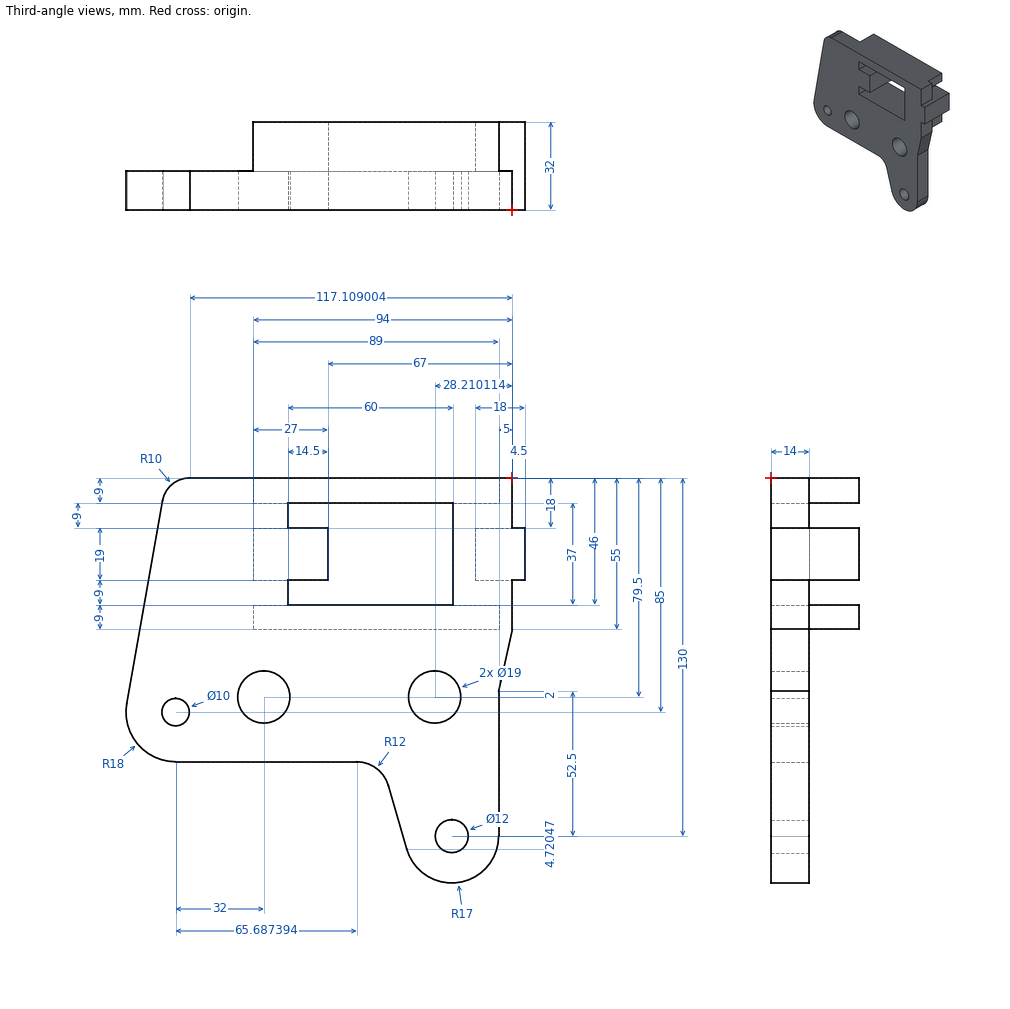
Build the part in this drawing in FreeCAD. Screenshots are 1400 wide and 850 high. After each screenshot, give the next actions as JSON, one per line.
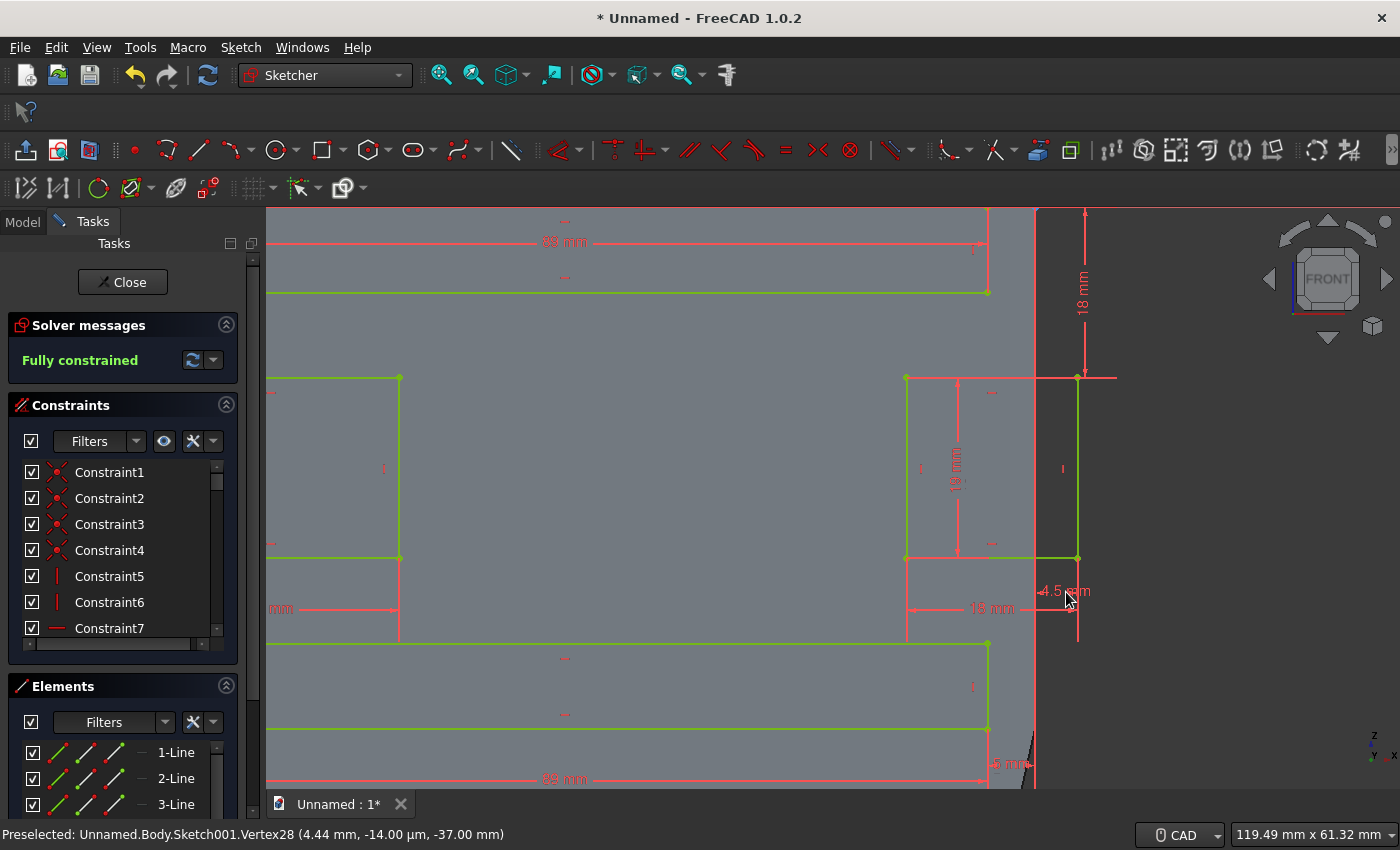
{"action": "left_click", "coordinate": [123, 282]}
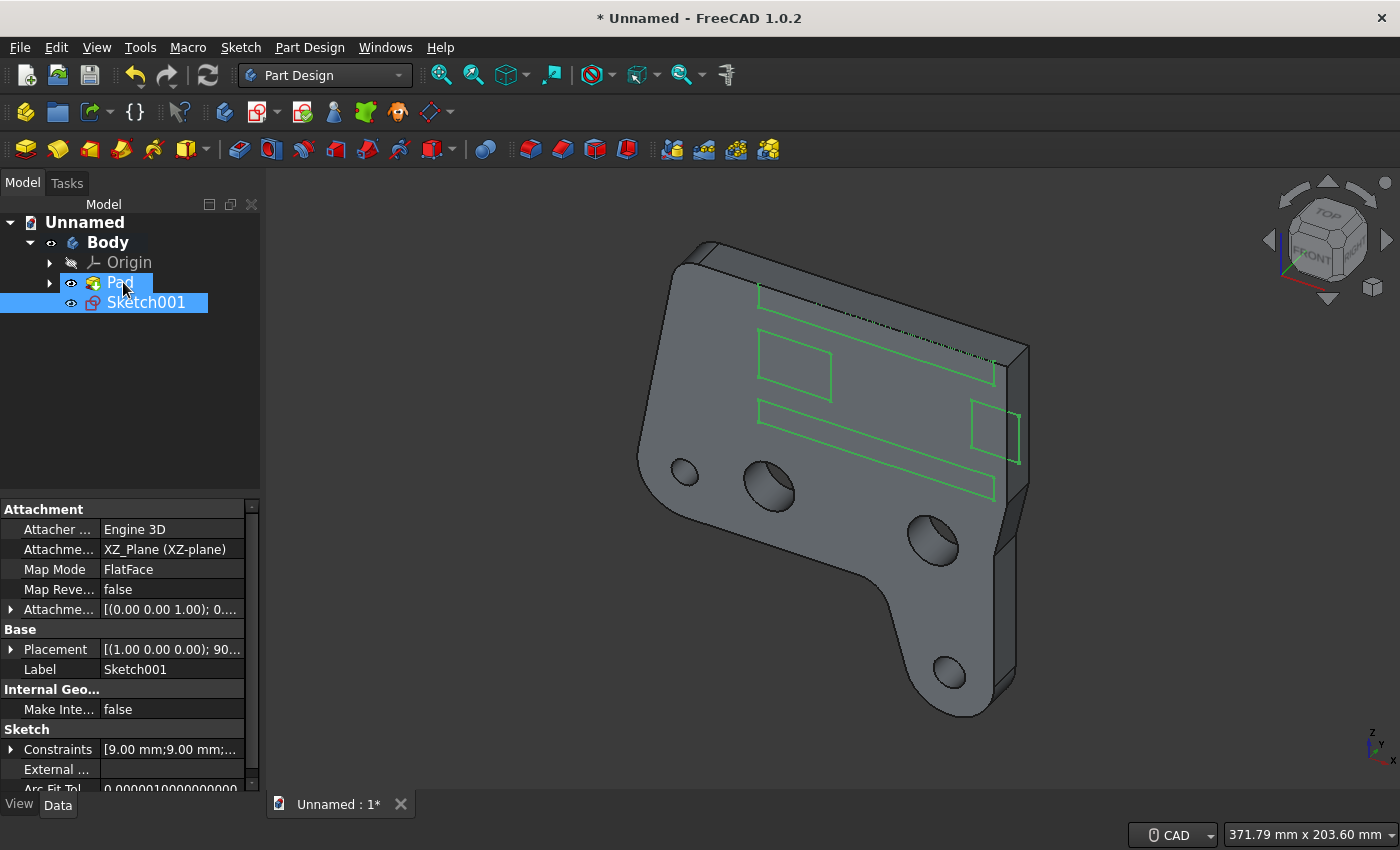
{"action": "left_click", "coordinate": [26, 150]}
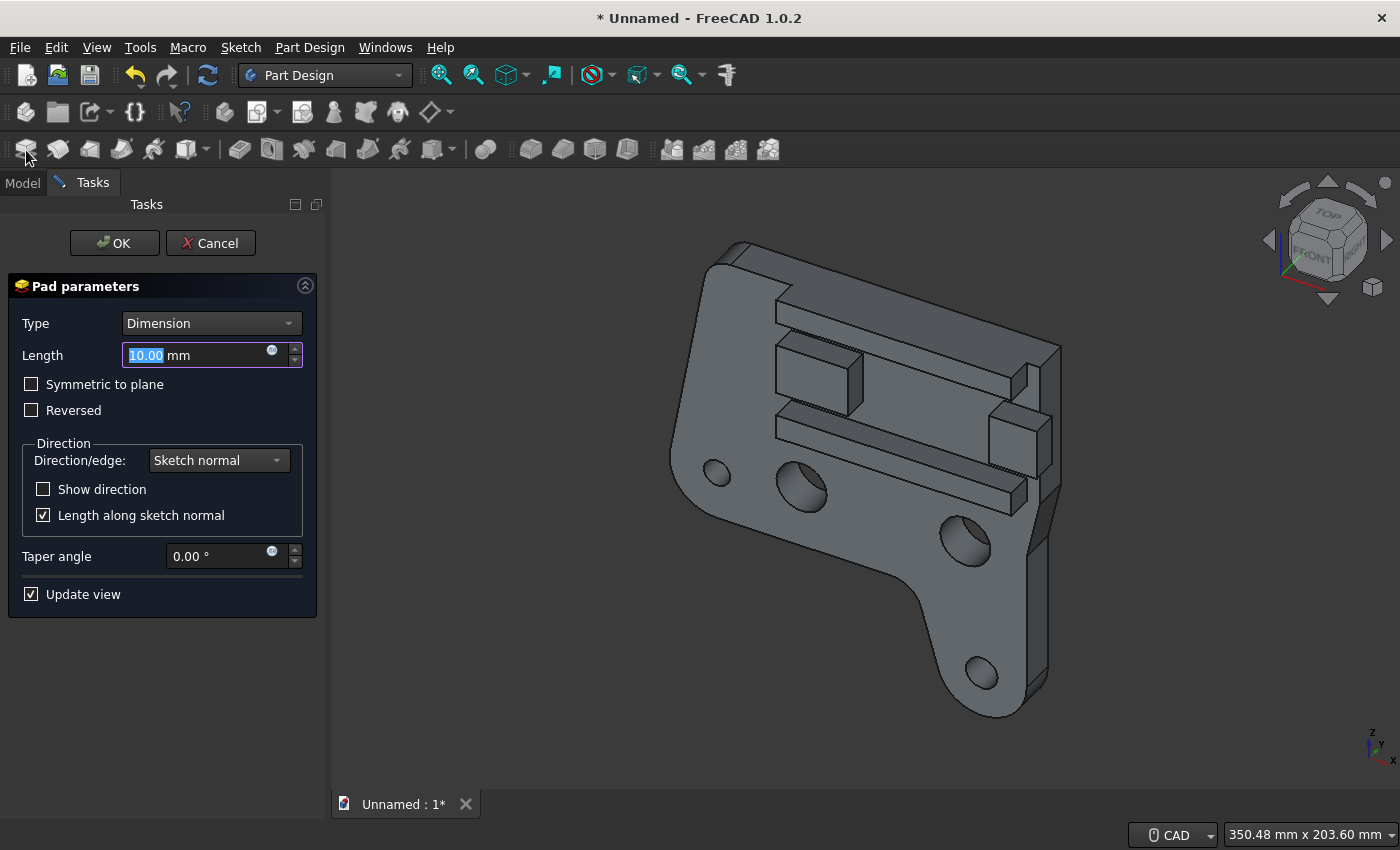
{"action": "type", "text": "32"}
{"action": "key", "text": "Tab"}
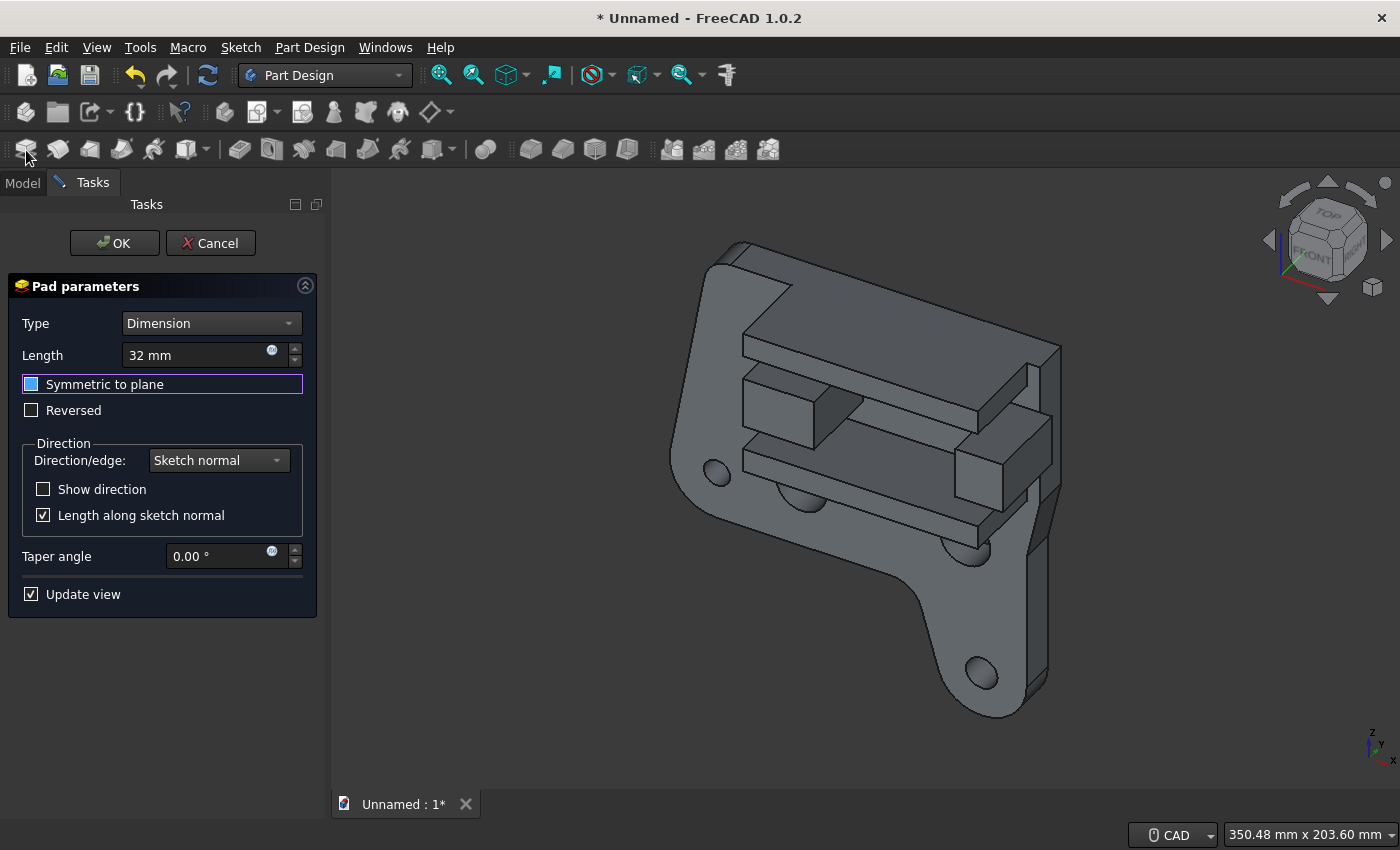
{"action": "left_click", "coordinate": [30, 410]}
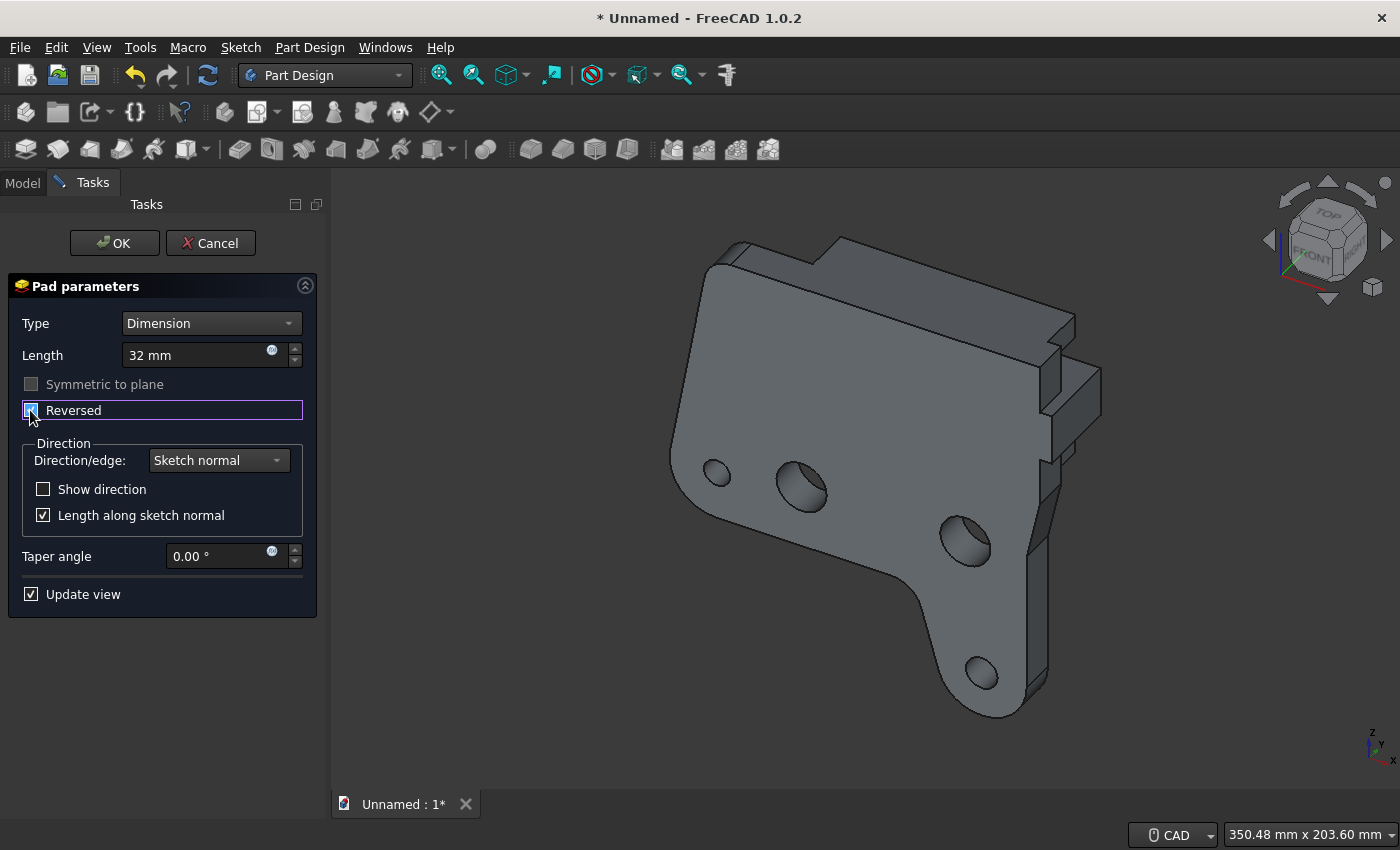
{"action": "left_click", "coordinate": [115, 243]}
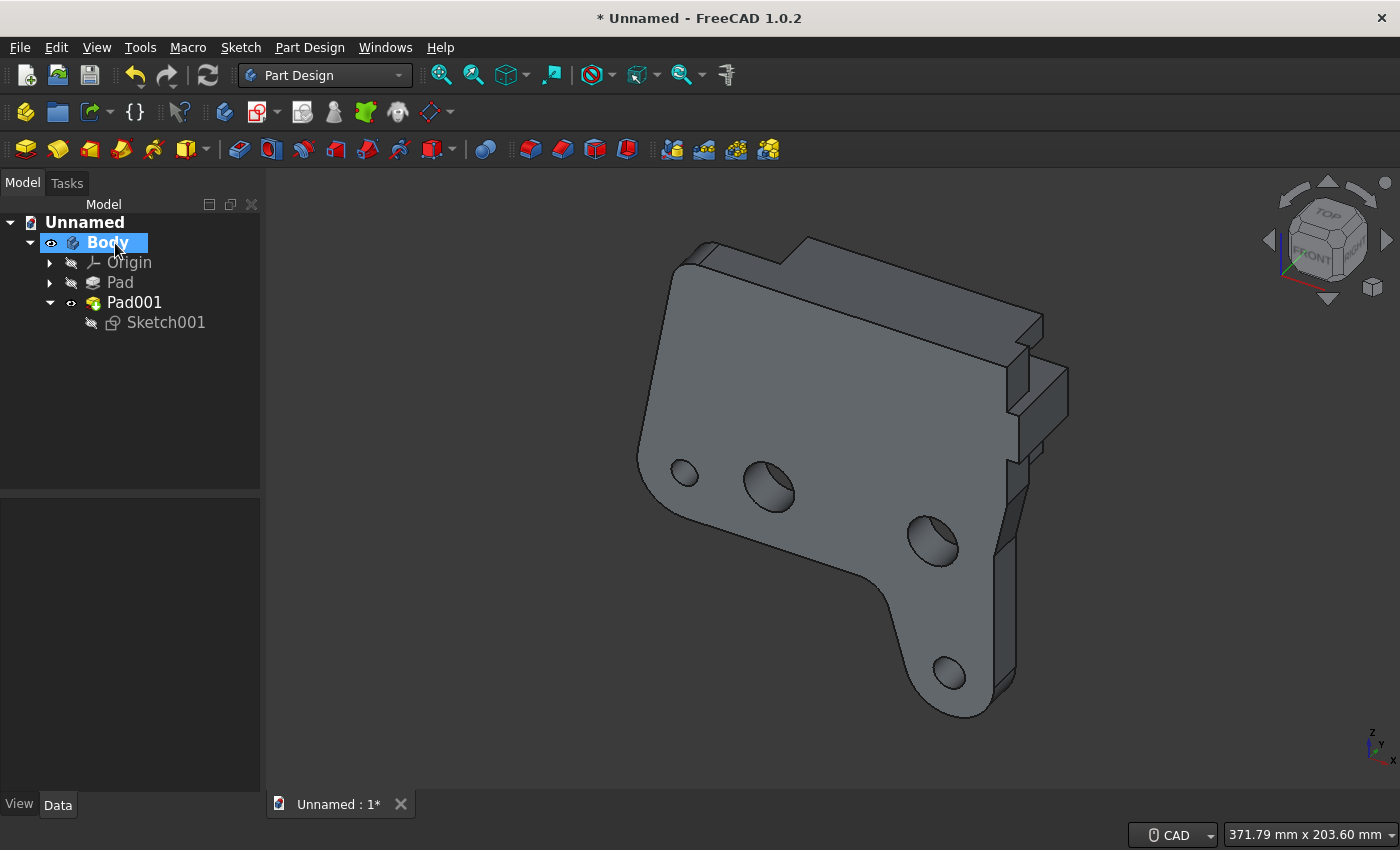
{"action": "key", "text": "4"}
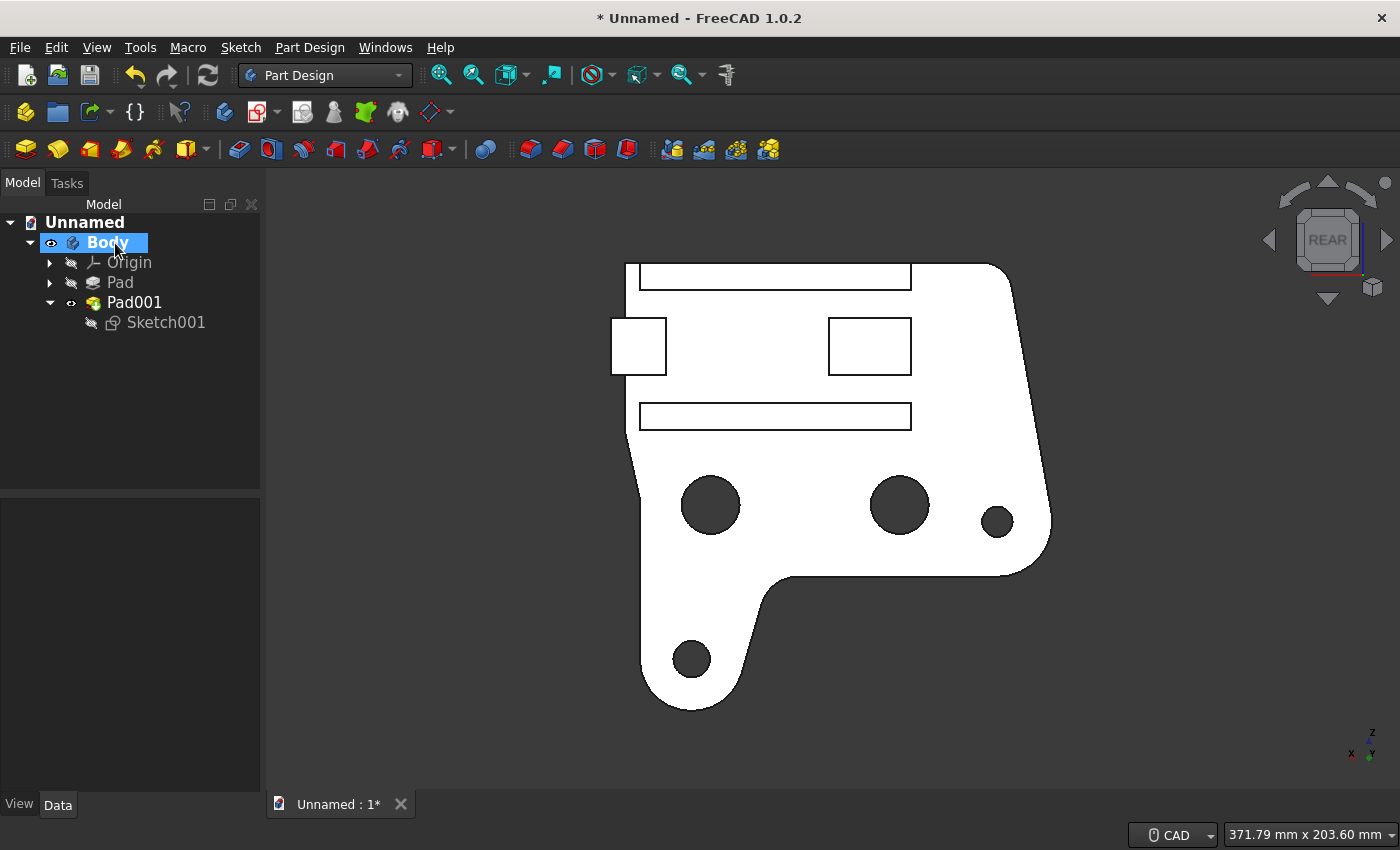
{"action": "left_click", "coordinate": [961, 358]}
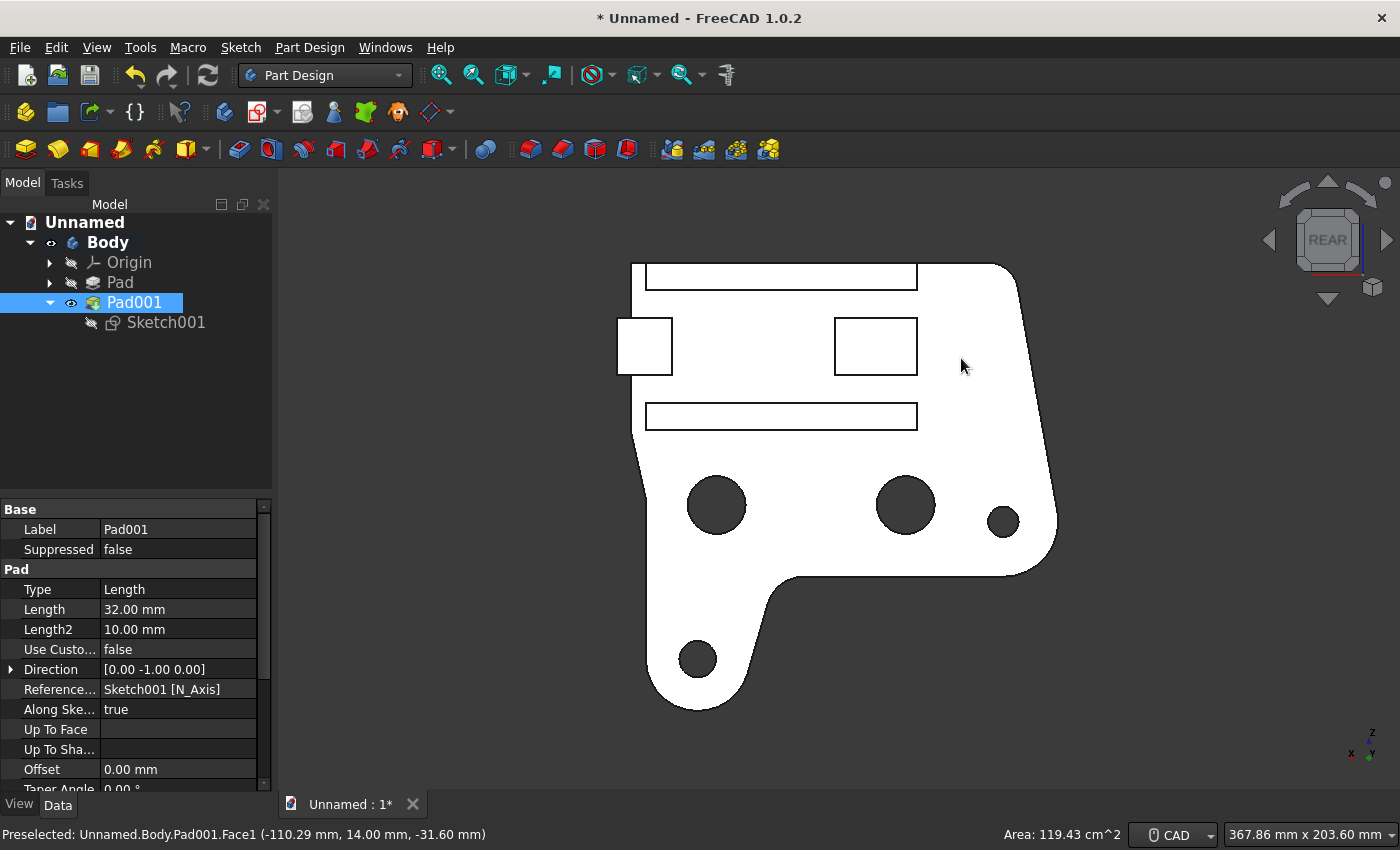
{"action": "left_click", "coordinate": [258, 112]}